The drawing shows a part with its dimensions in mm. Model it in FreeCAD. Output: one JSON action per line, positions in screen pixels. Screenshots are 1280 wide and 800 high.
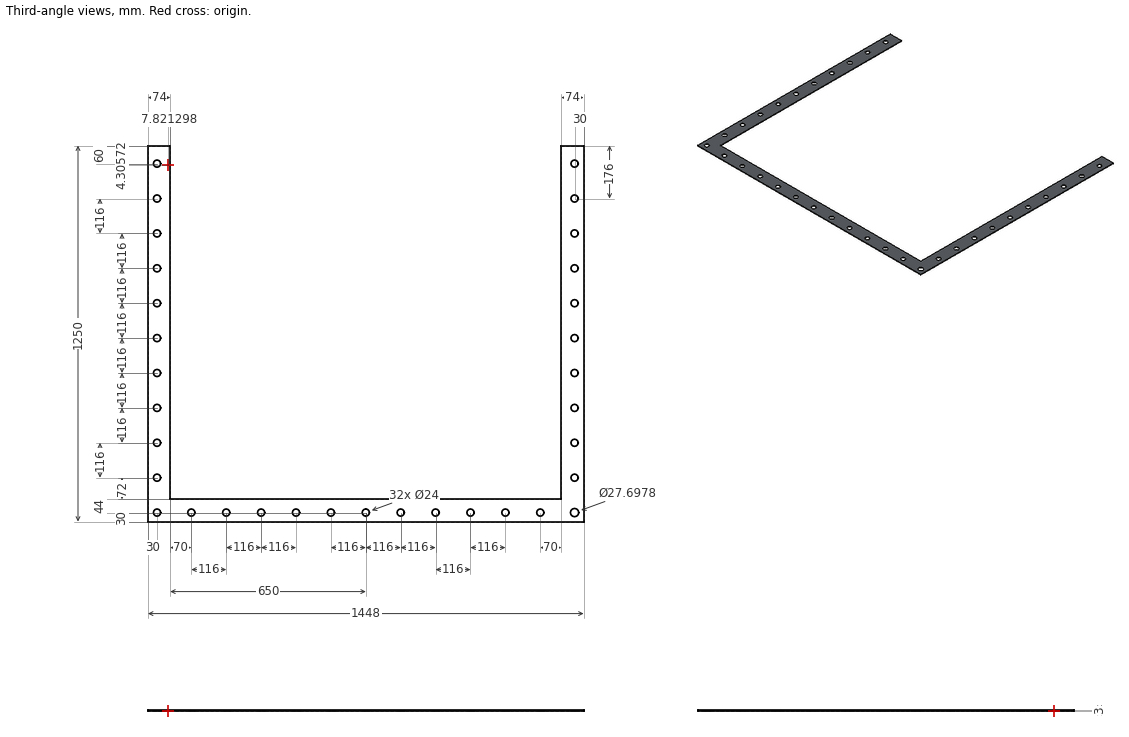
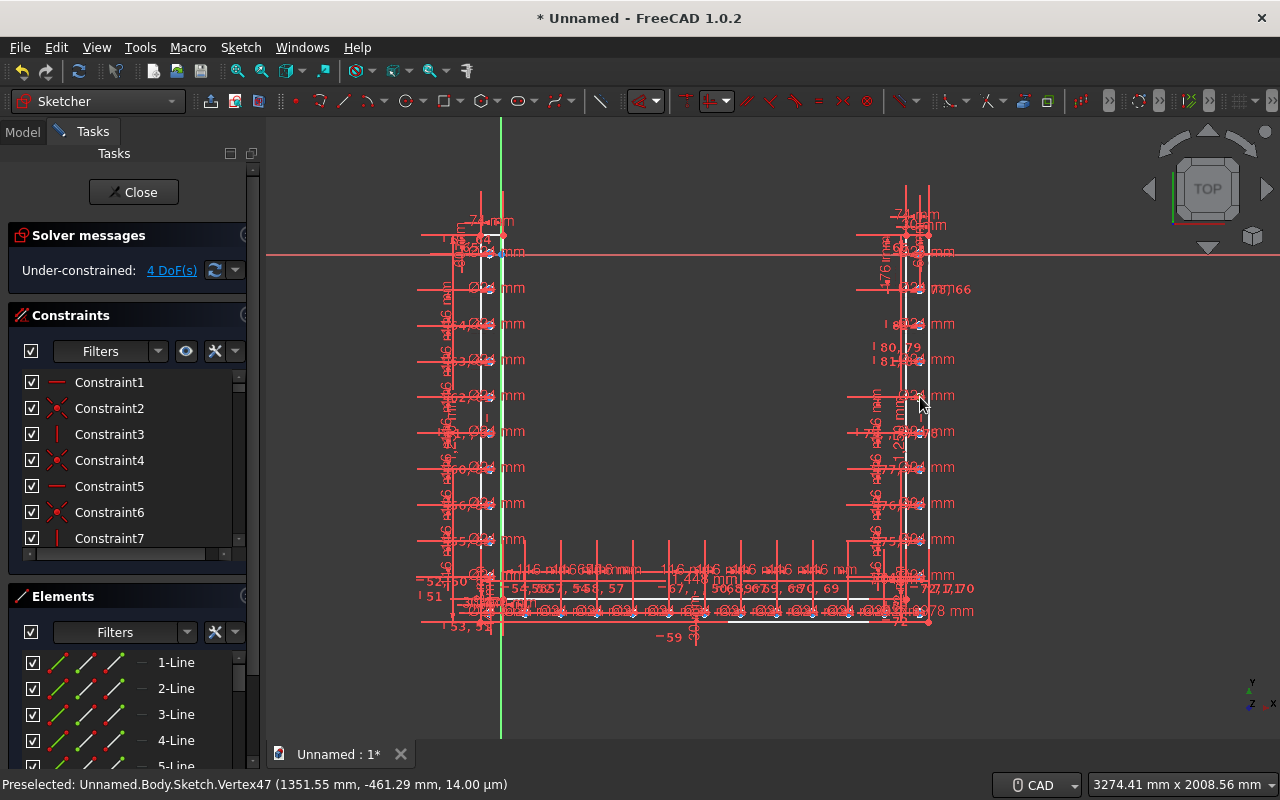
{"action": "left_click", "coordinate": [920, 361]}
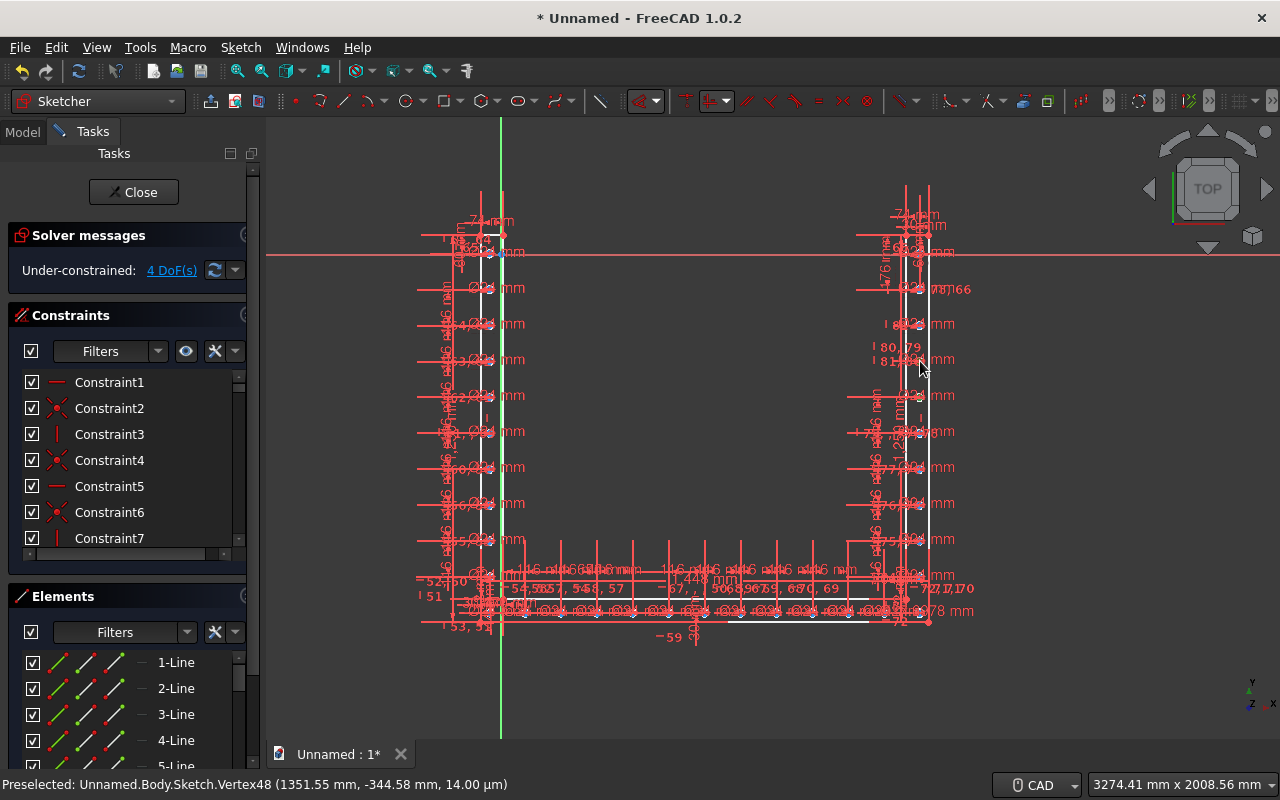
{"action": "left_click", "coordinate": [658, 102]}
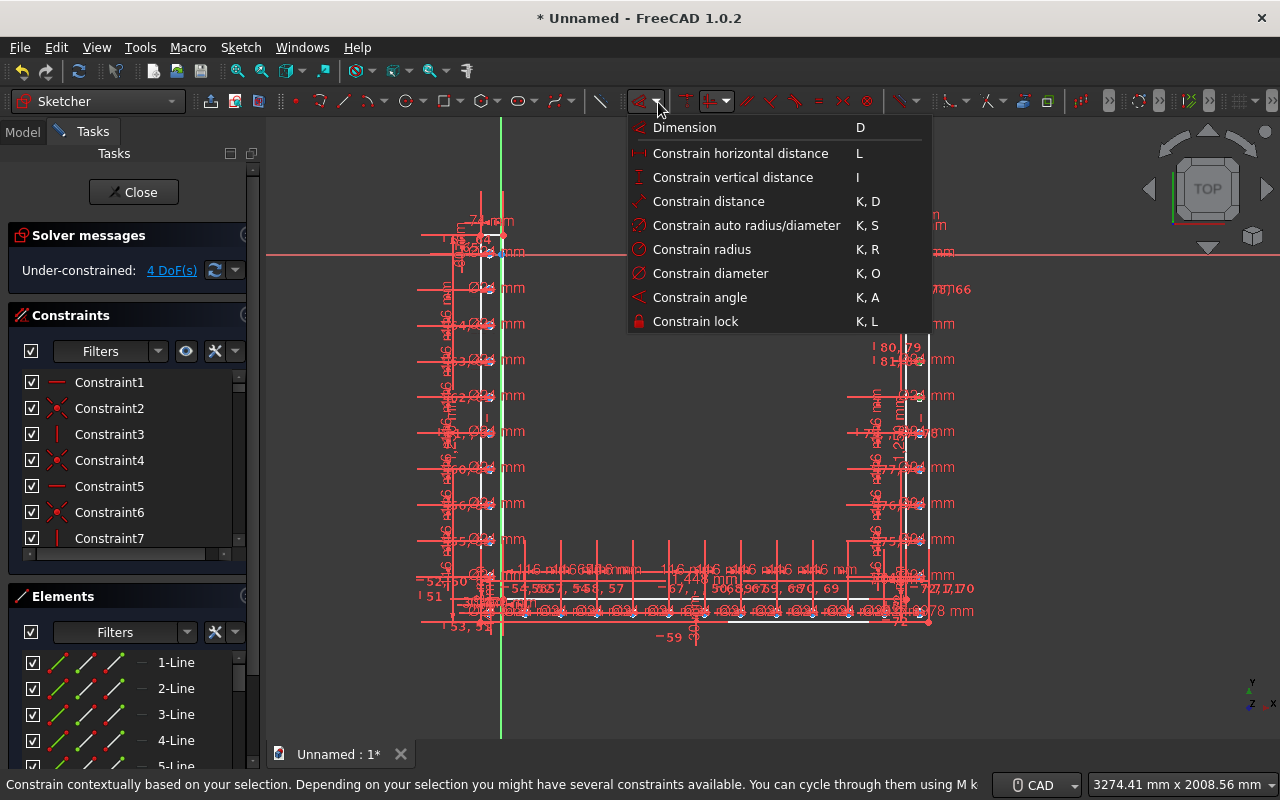
{"action": "left_click", "coordinate": [780, 177]}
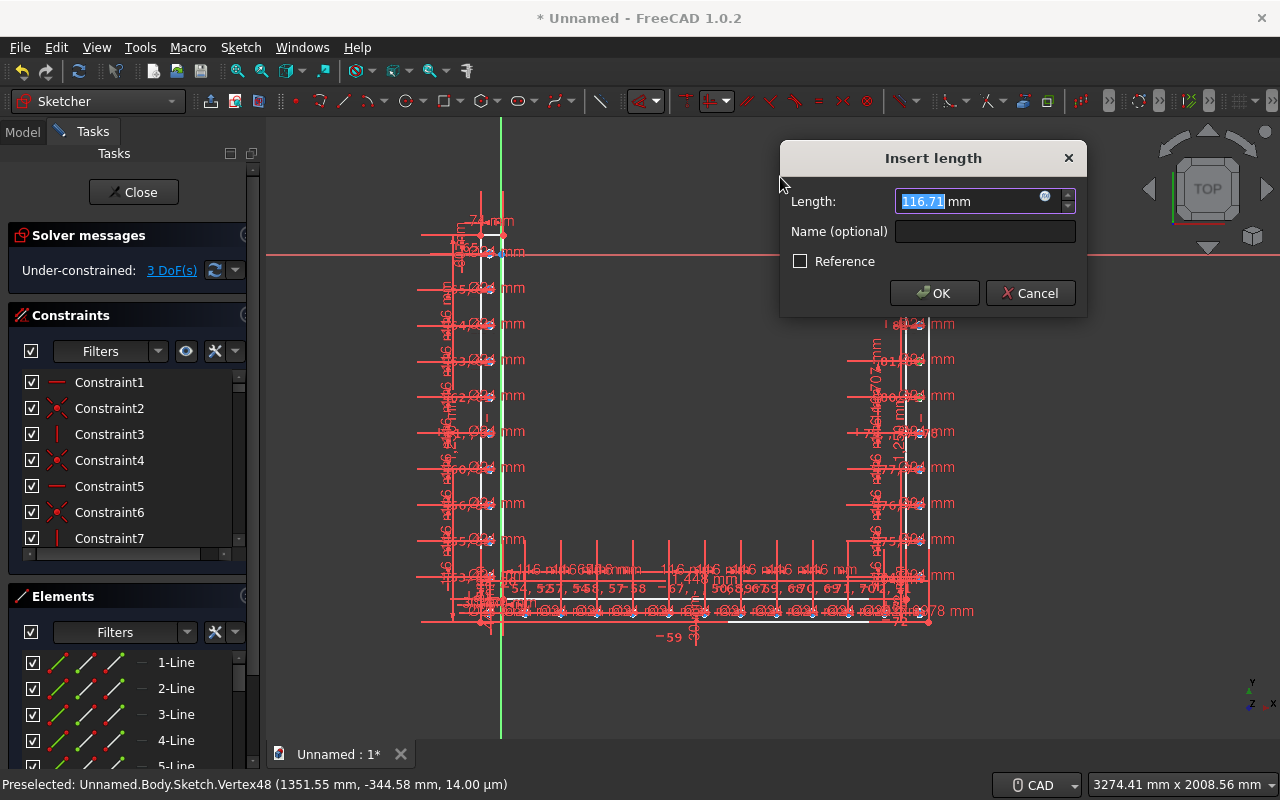
{"action": "type", "text": "116"}
{"action": "key", "text": "Return"}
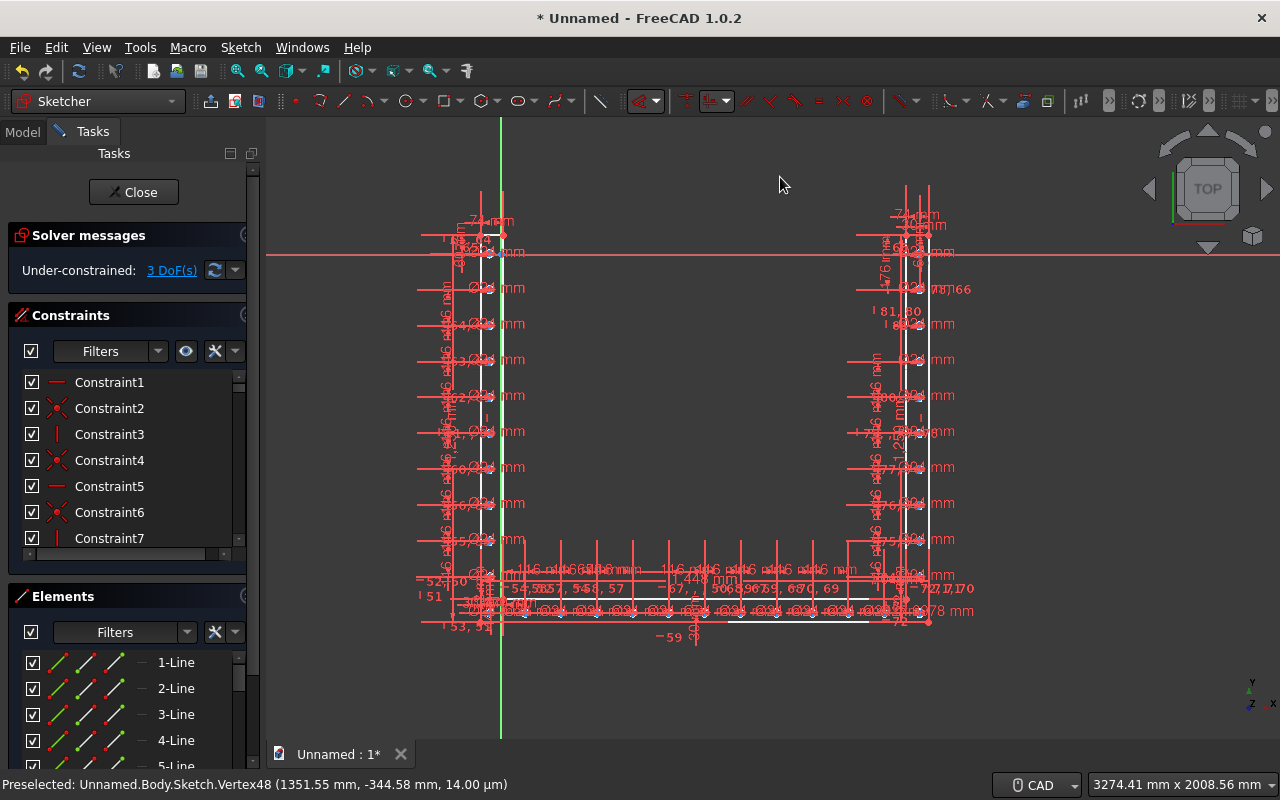
{"action": "left_click", "coordinate": [920, 362]}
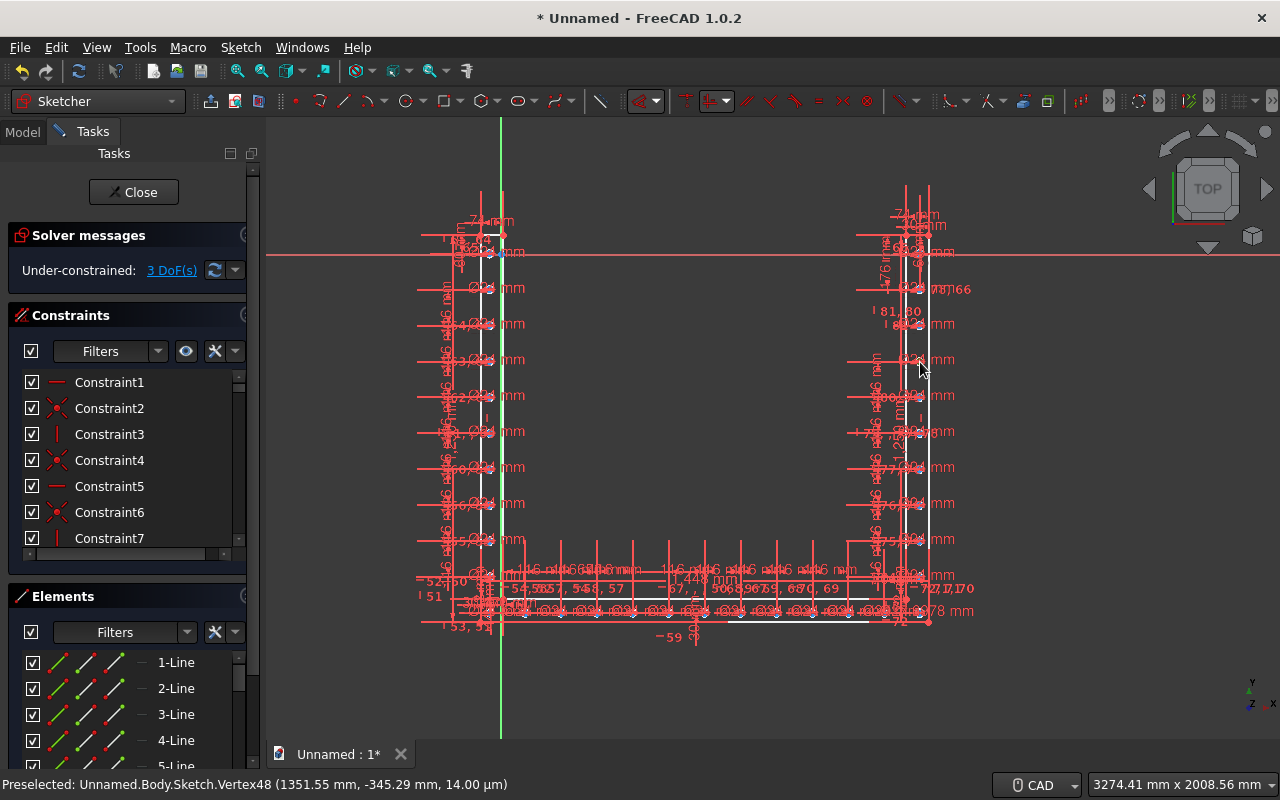
{"action": "left_click", "coordinate": [920, 326]}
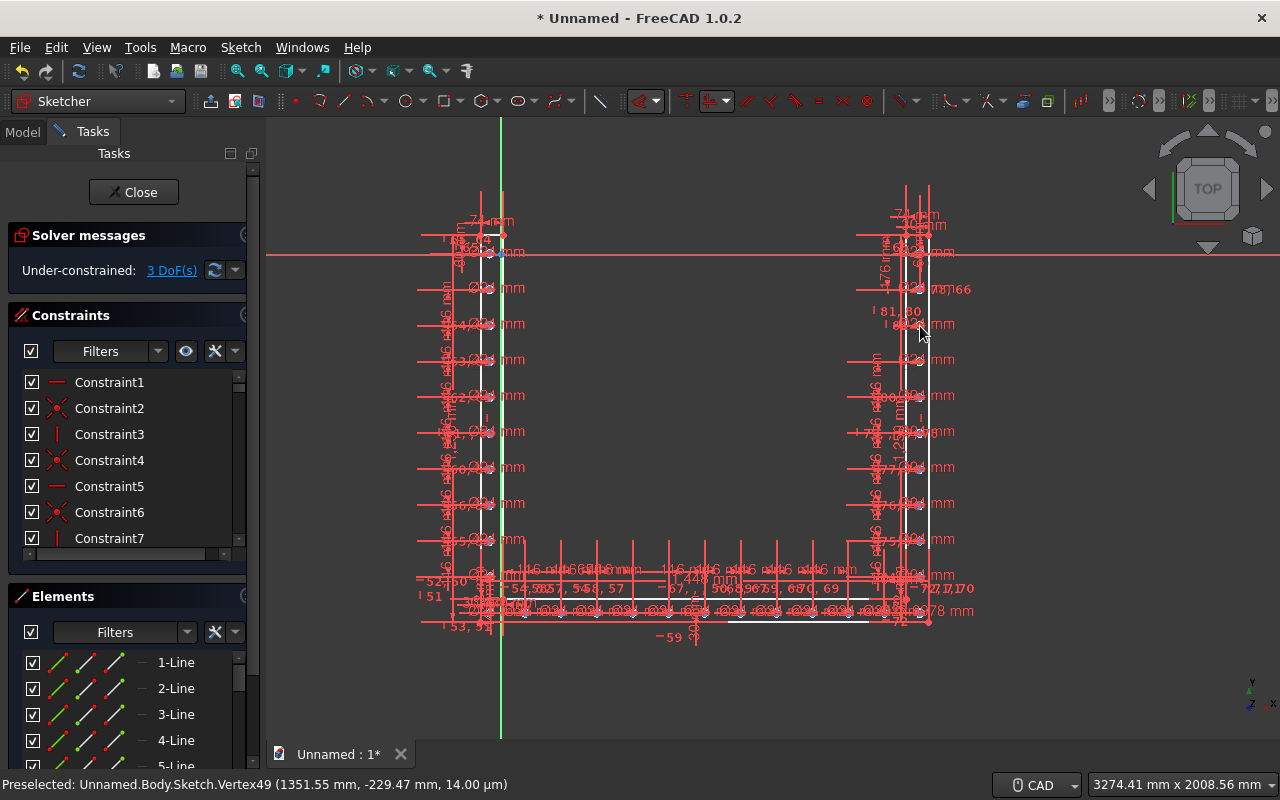
{"action": "left_click", "coordinate": [658, 102]}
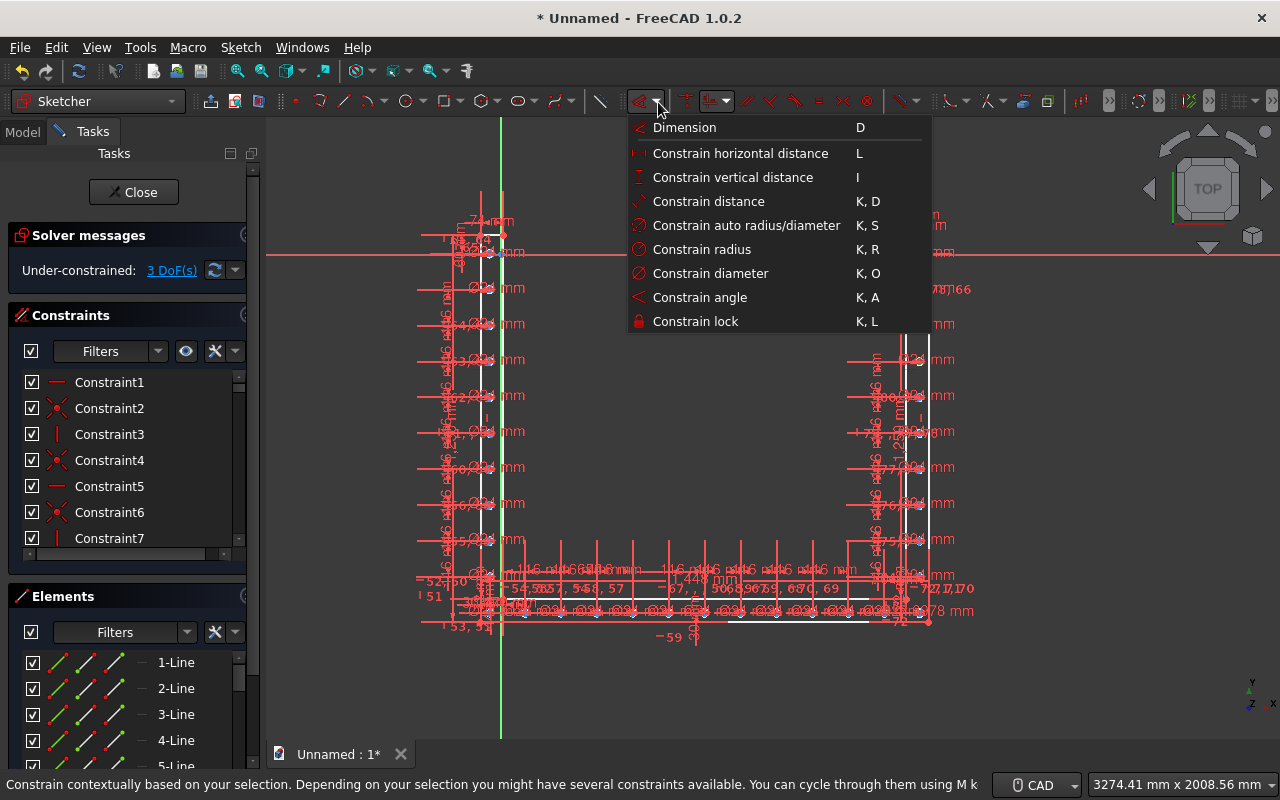
{"action": "left_click", "coordinate": [780, 177]}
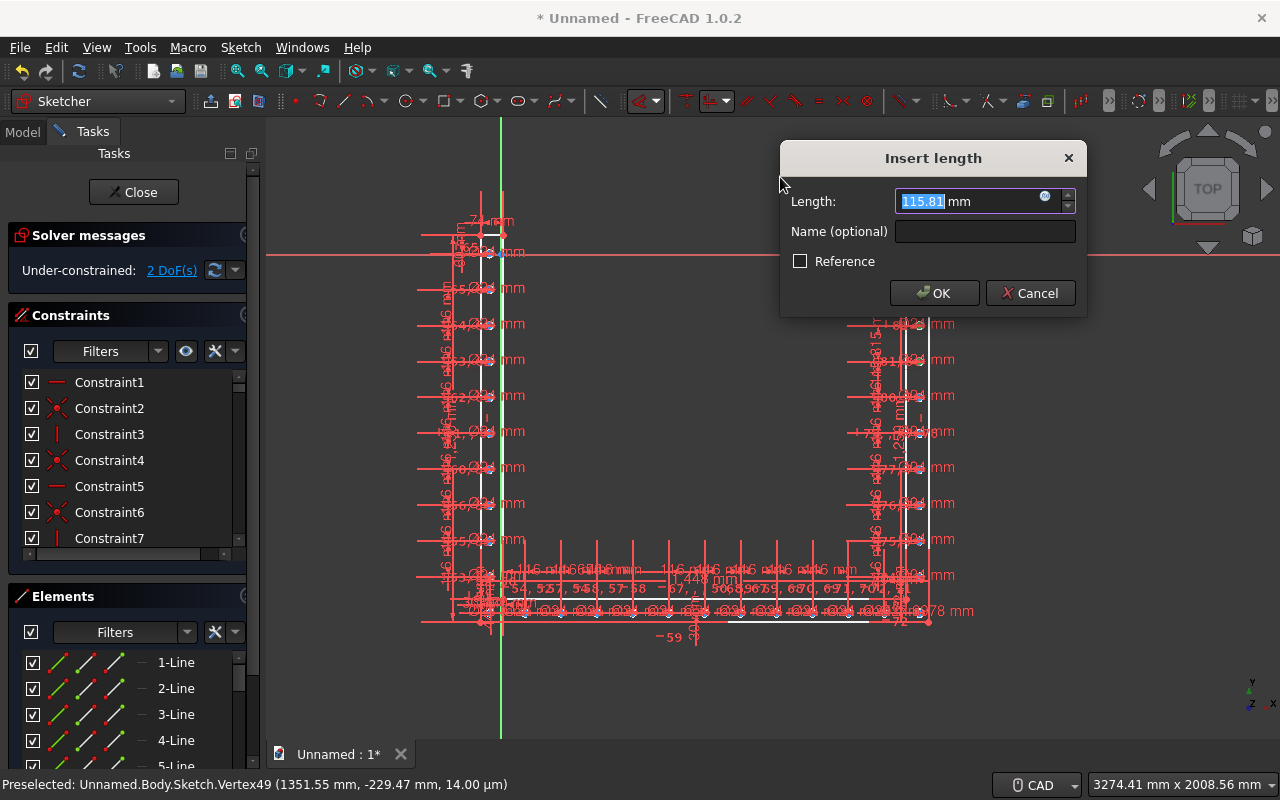
{"action": "type", "text": "116"}
{"action": "key", "text": "Return"}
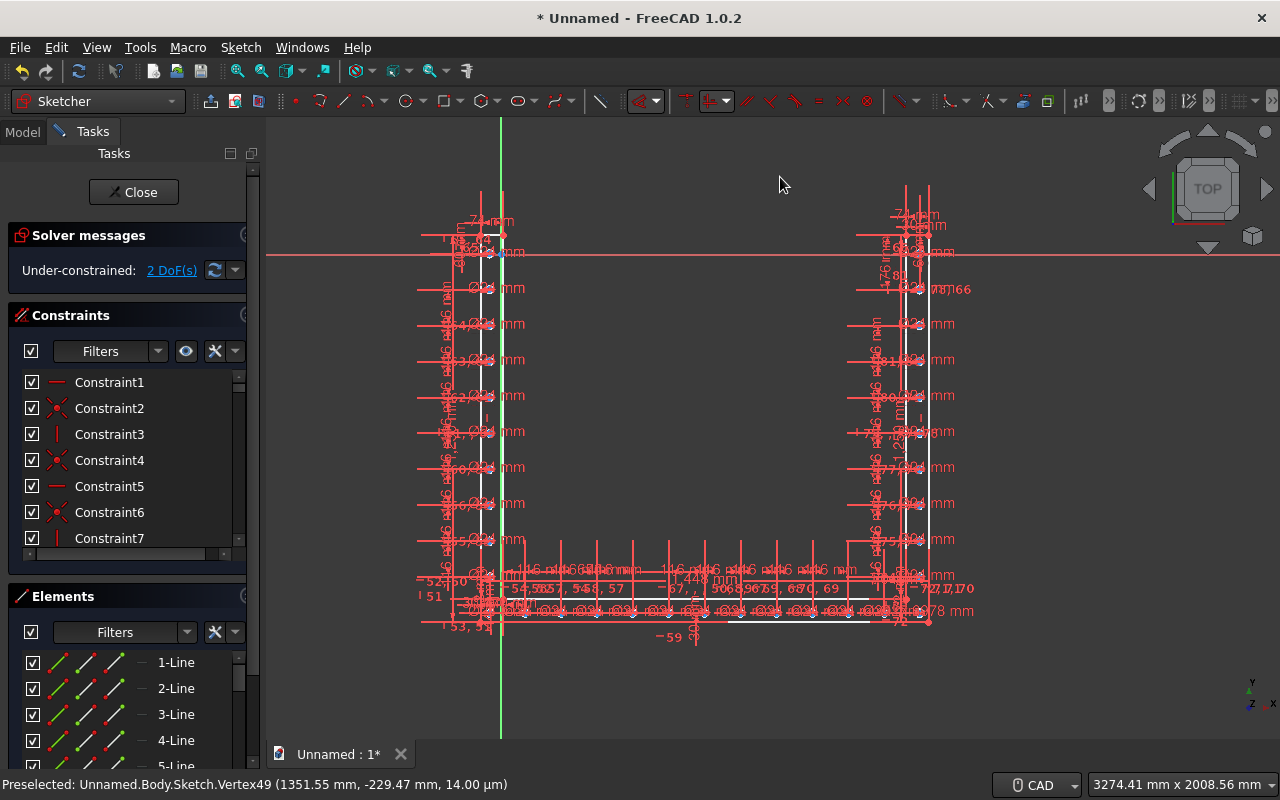
{"action": "scroll", "coordinate": [490, 254], "scroll_direction": "up", "scroll_amount": 17}